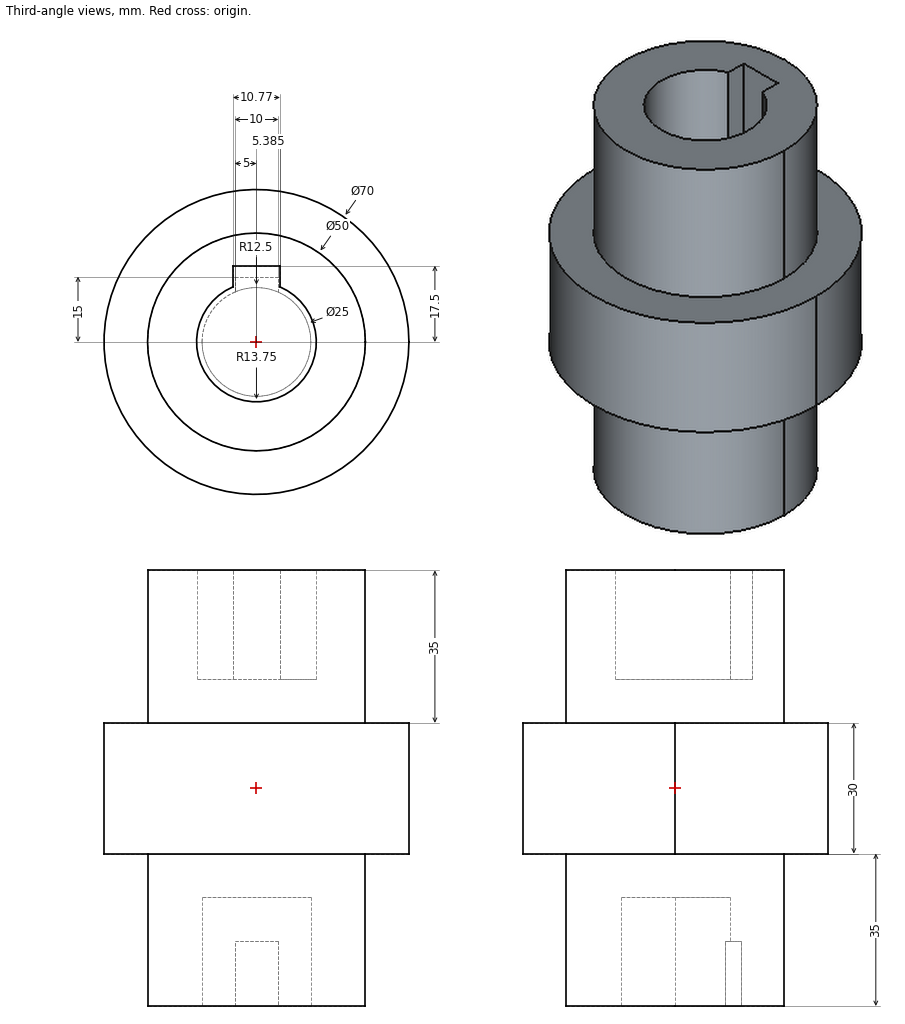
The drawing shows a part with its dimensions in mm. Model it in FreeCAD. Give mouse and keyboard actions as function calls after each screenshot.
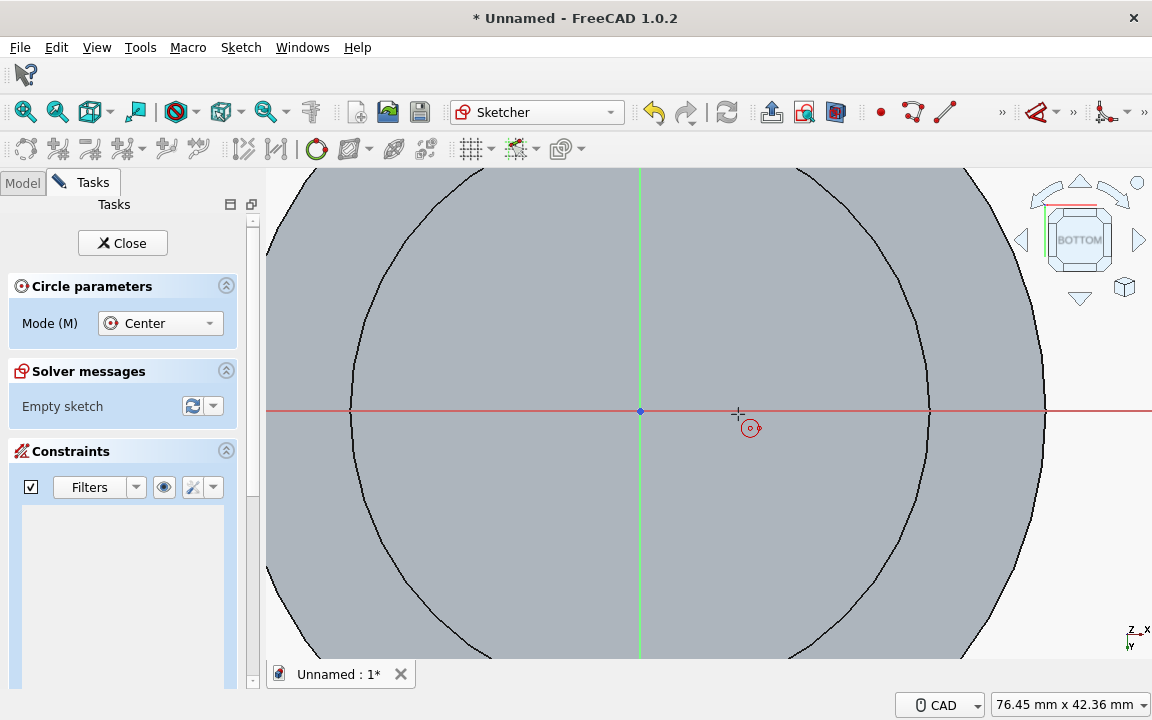
click(640, 411)
move(742, 309)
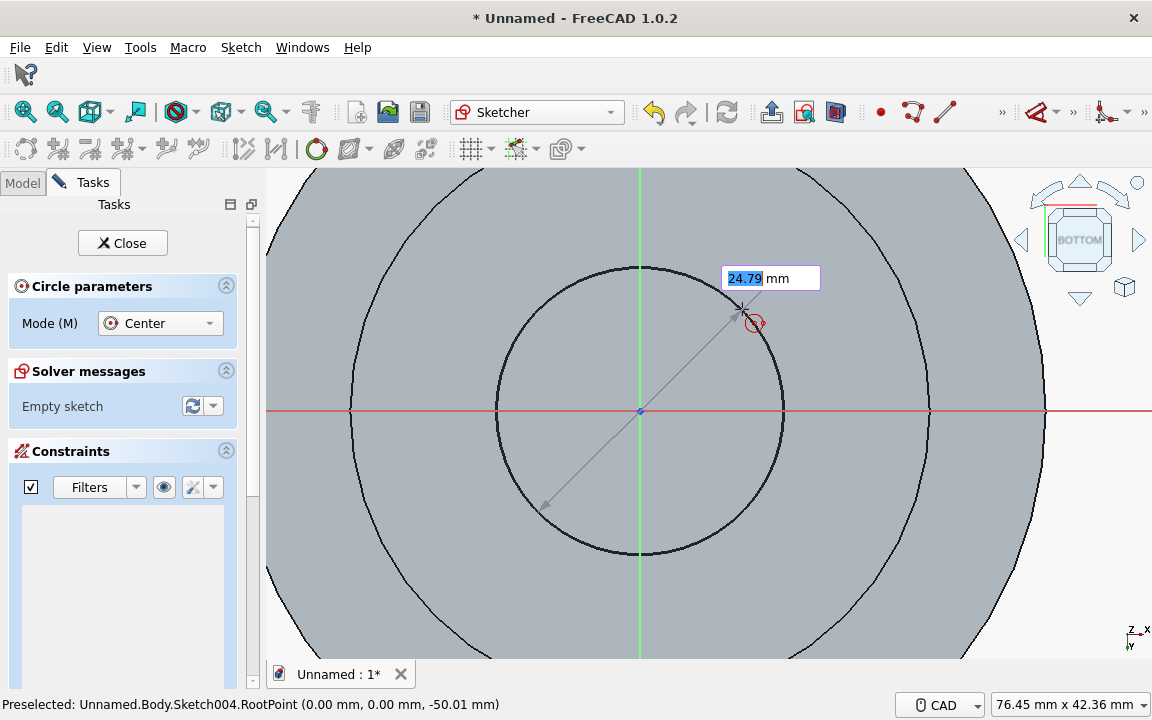
text(25)
key(Return)
key(Escape)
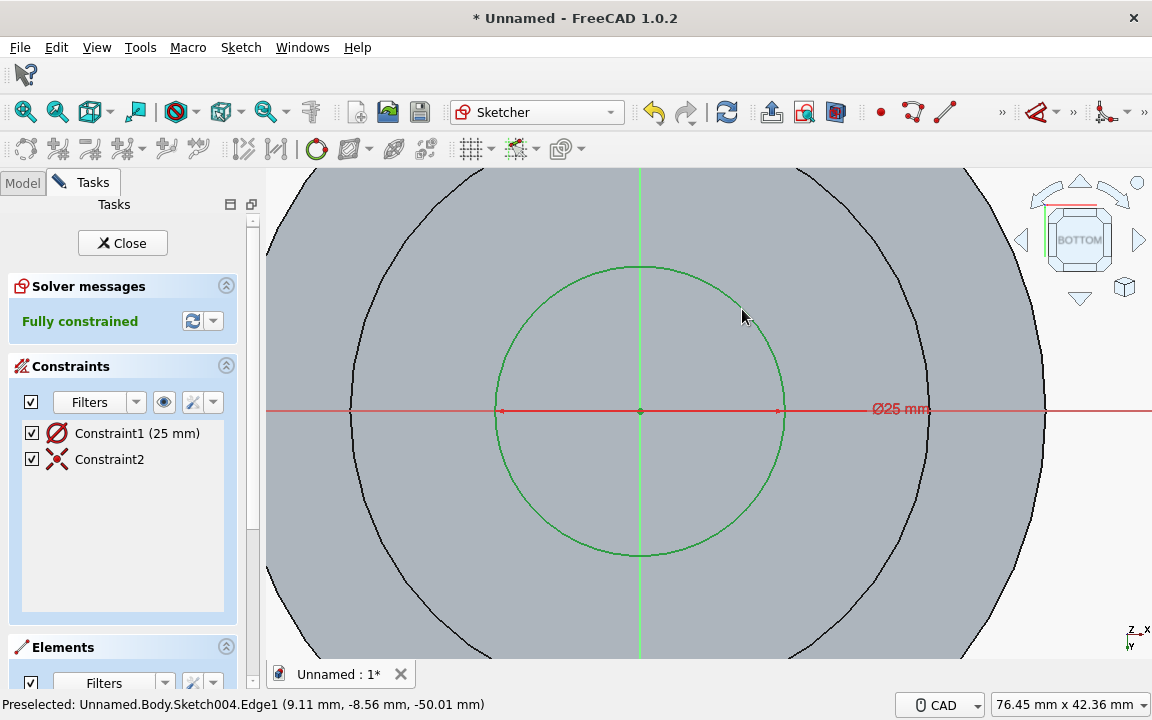
click(123, 243)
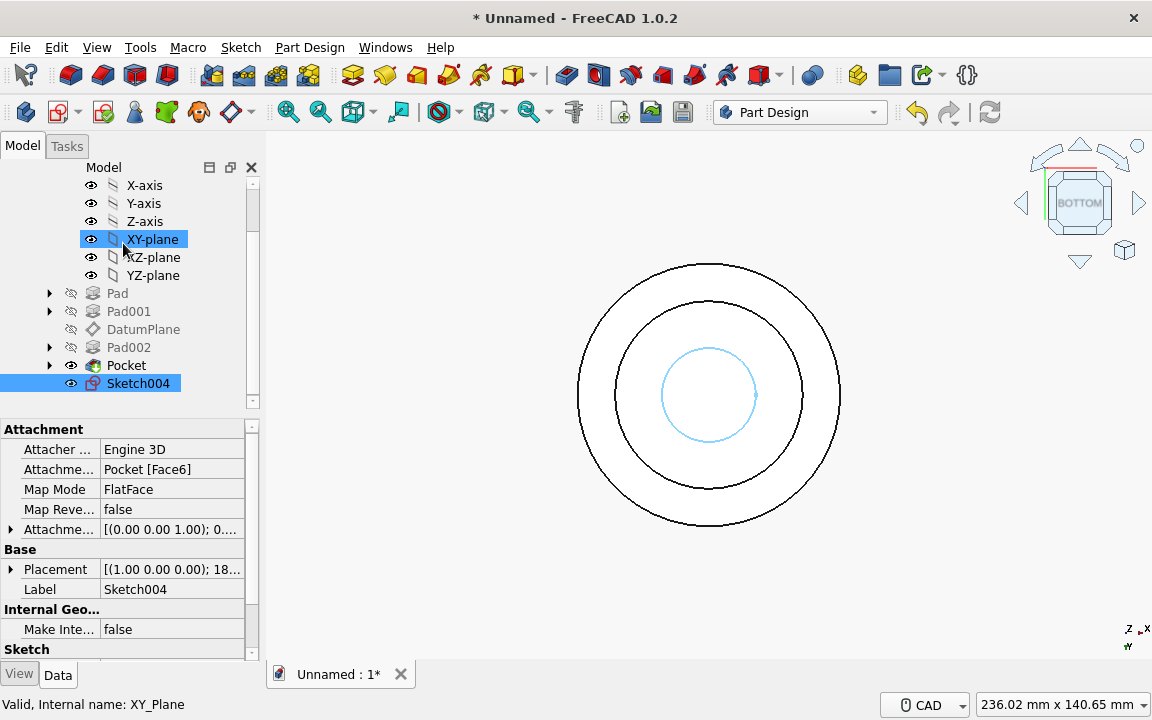
click(568, 76)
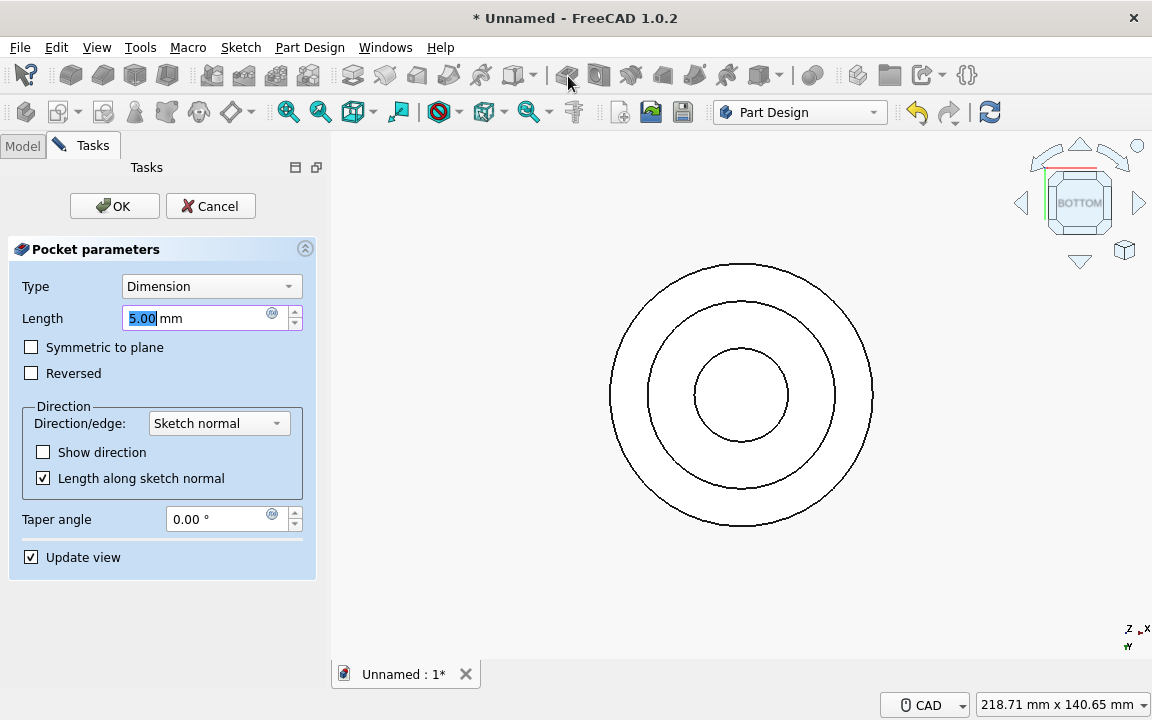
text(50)
key(Tab)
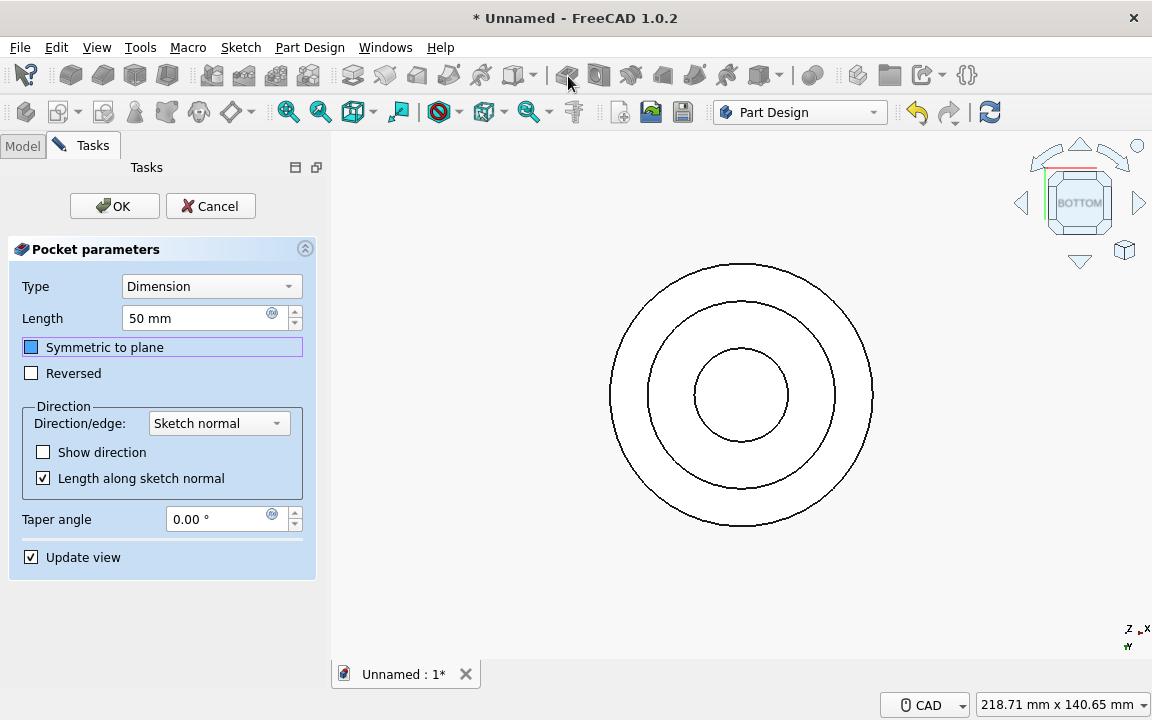
click(30, 347)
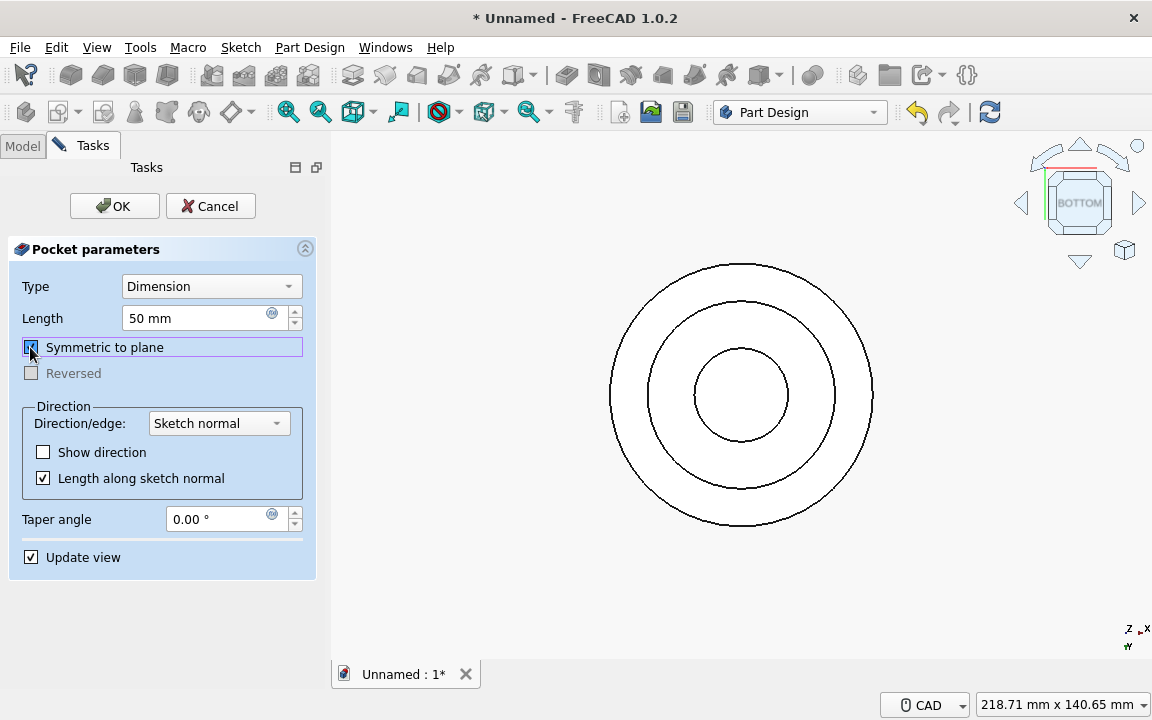
click(115, 206)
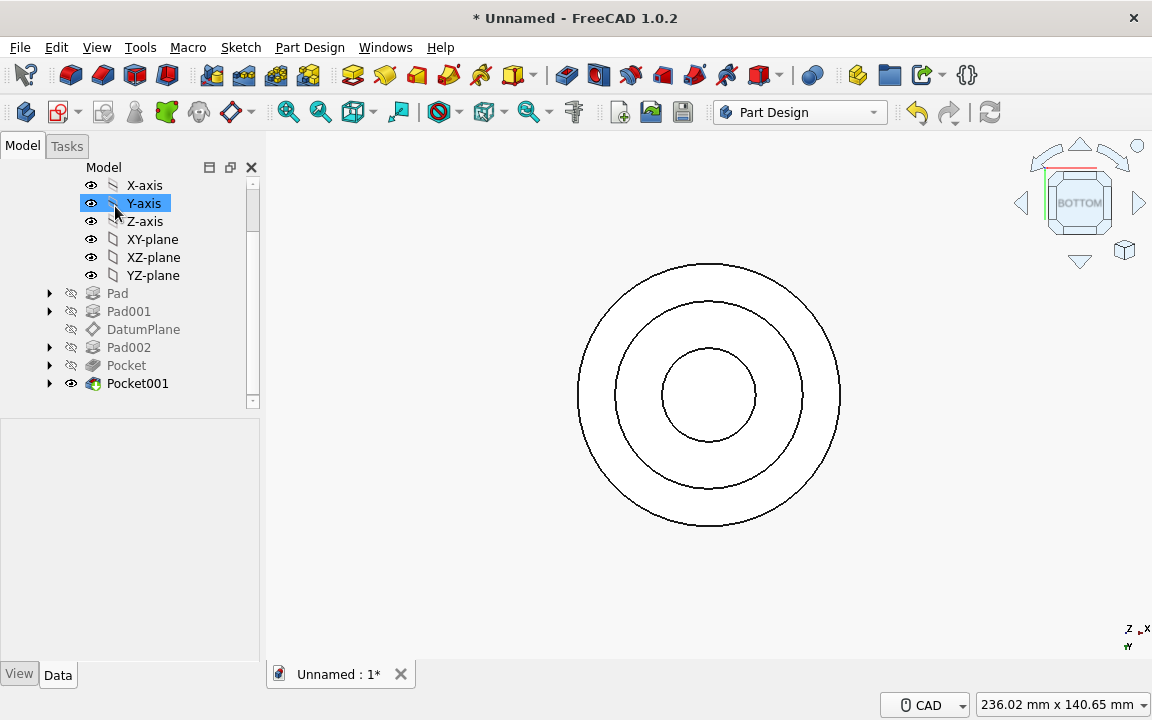
click(762, 340)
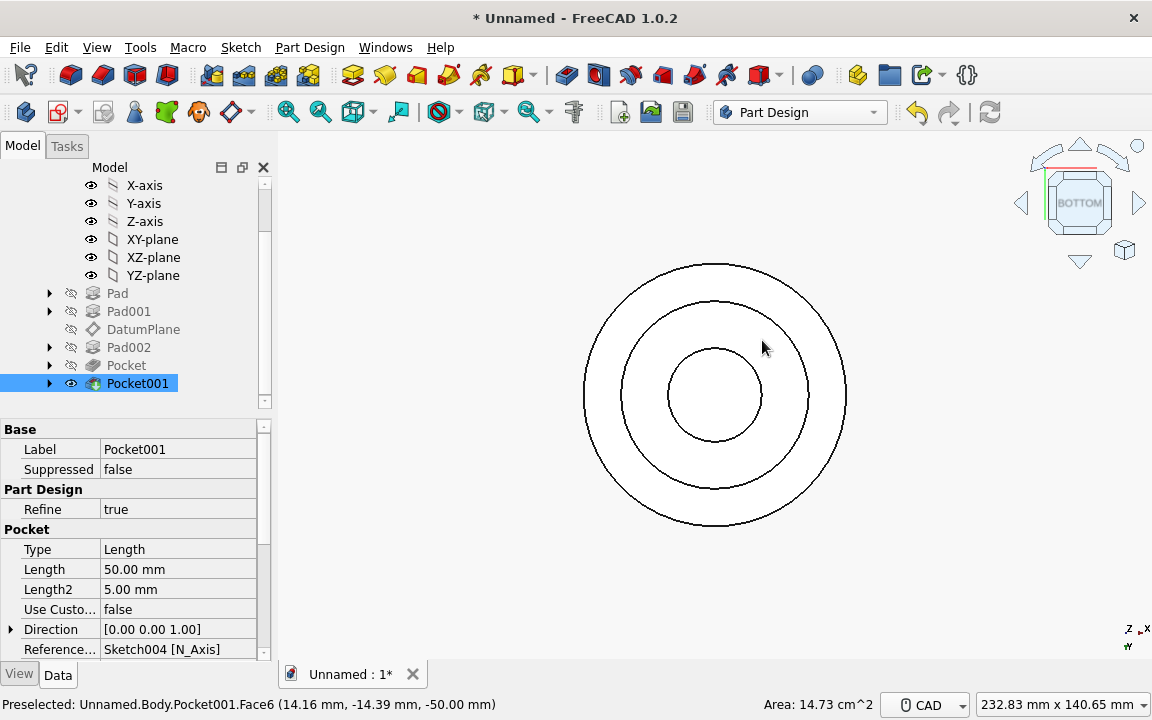
click(58, 112)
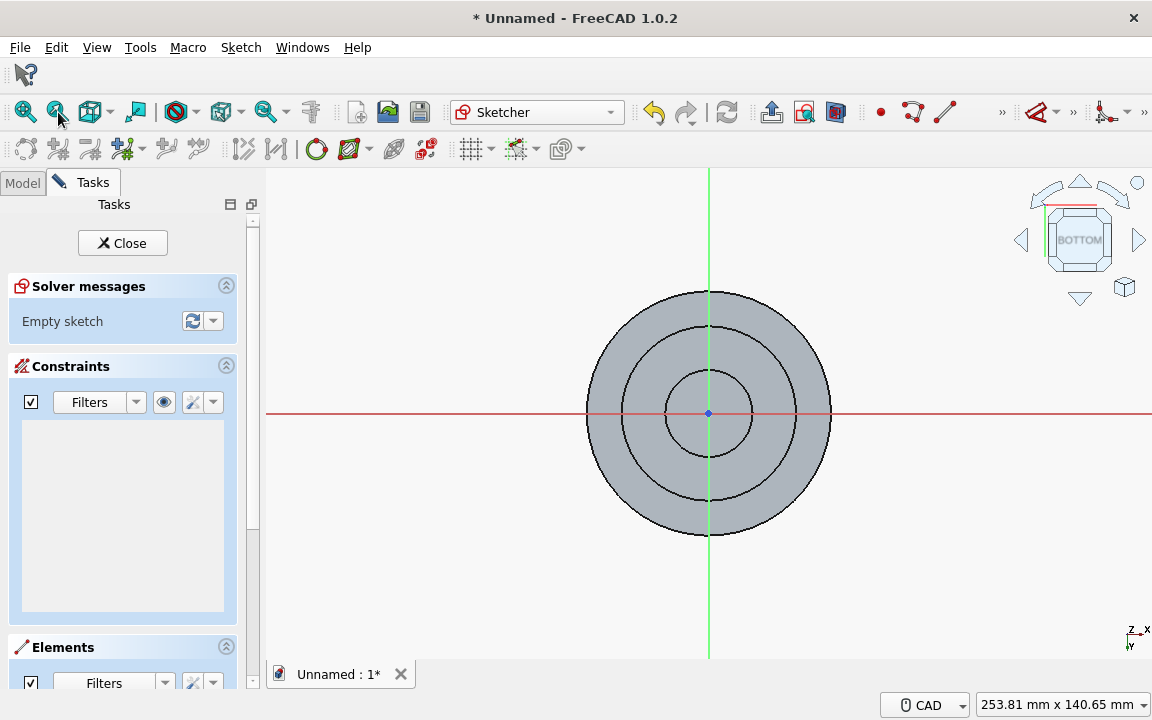
scroll(722, 445, up, 9)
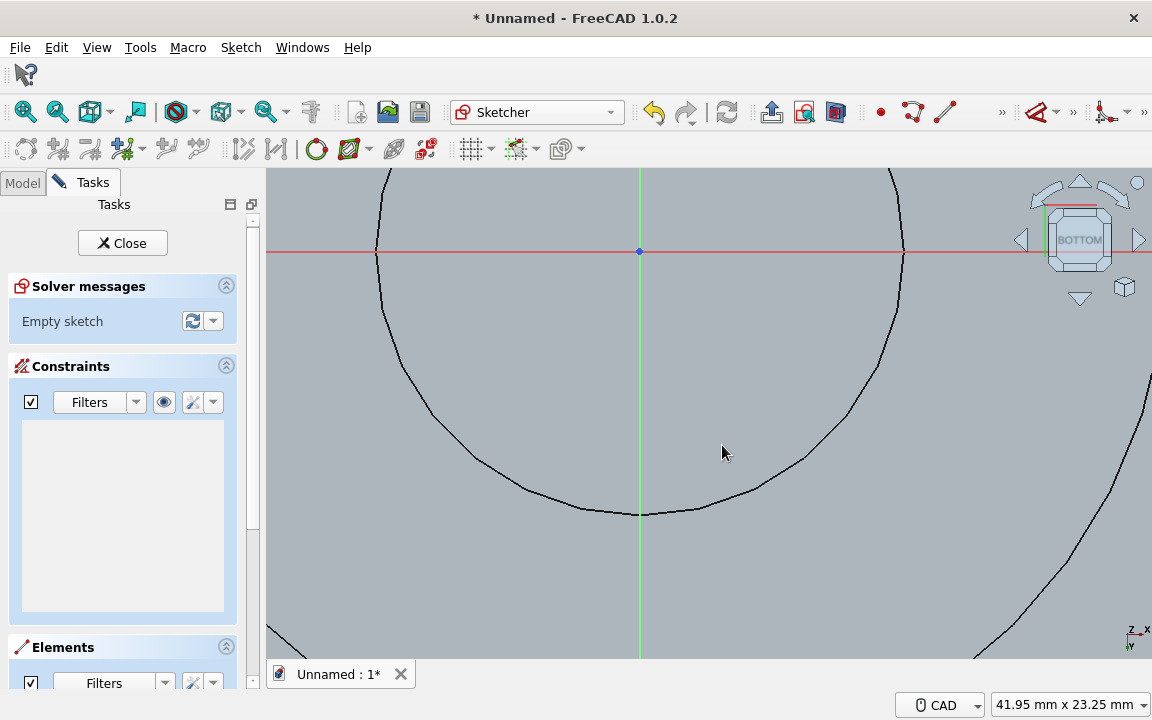
key(g)
key(m)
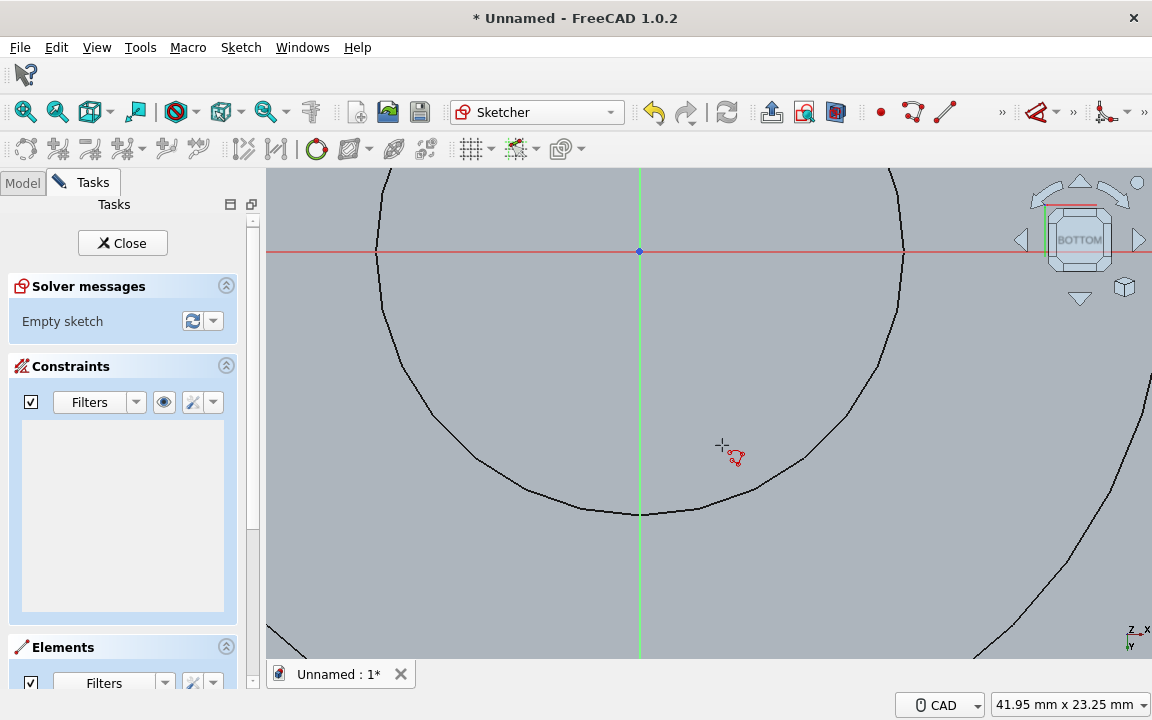
click(534, 494)
click(534, 568)
click(746, 568)
click(746, 494)
right_click(746, 494)